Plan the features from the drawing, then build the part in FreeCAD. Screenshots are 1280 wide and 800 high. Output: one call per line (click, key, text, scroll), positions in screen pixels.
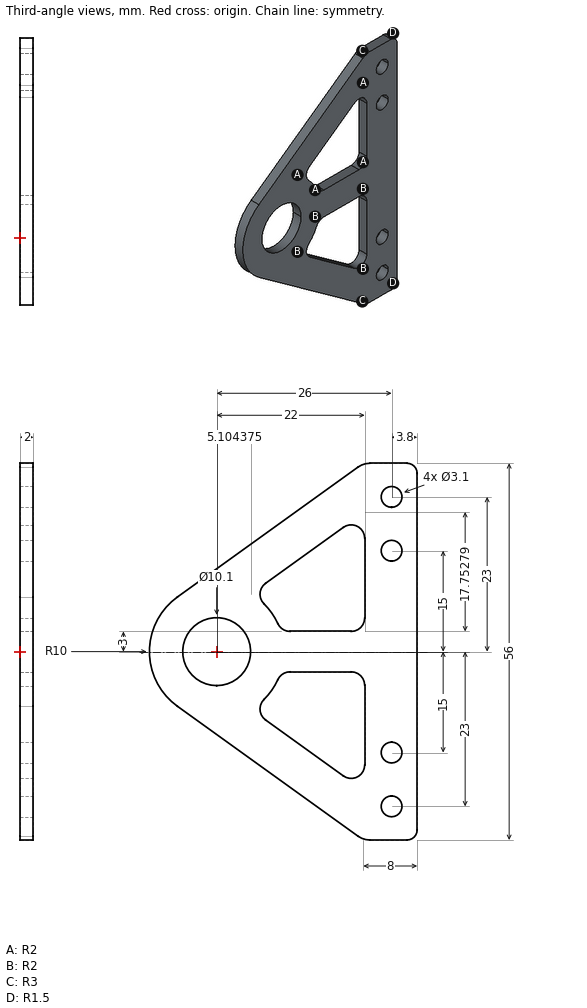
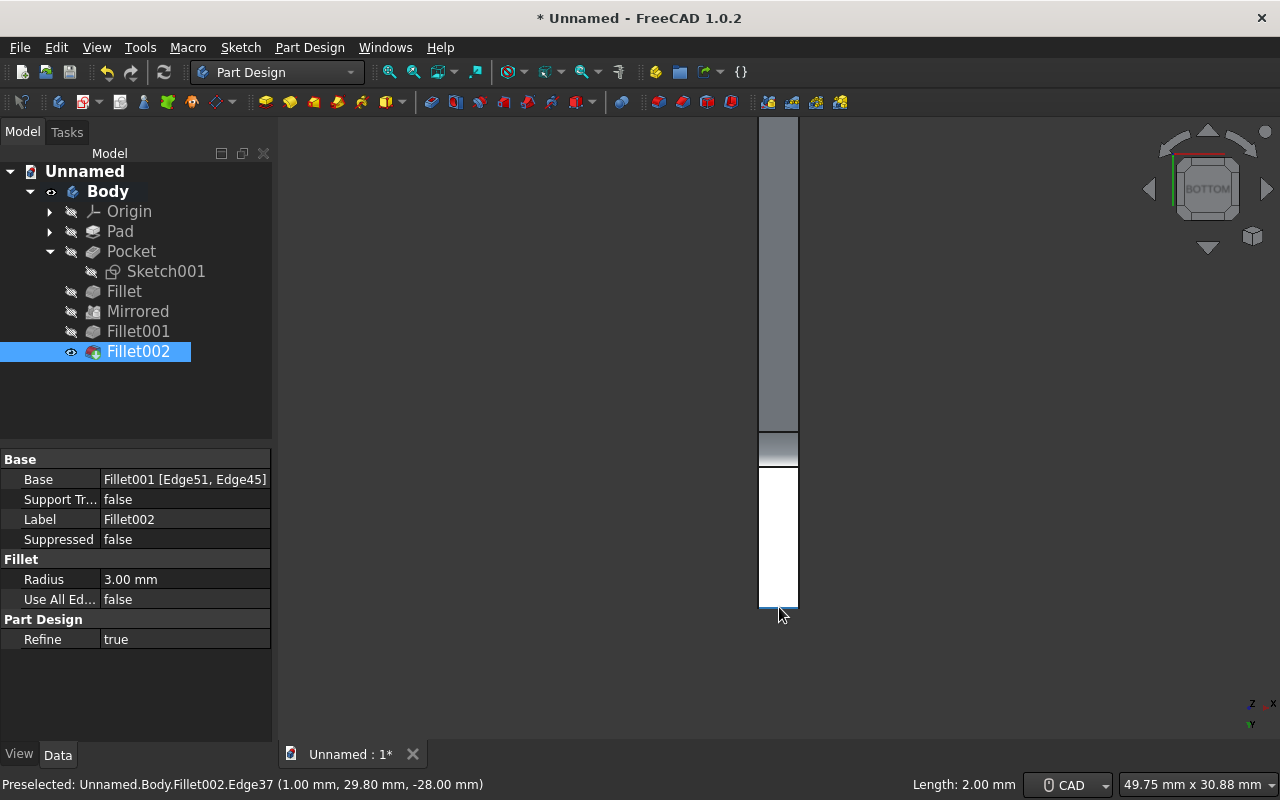
click(390, 72)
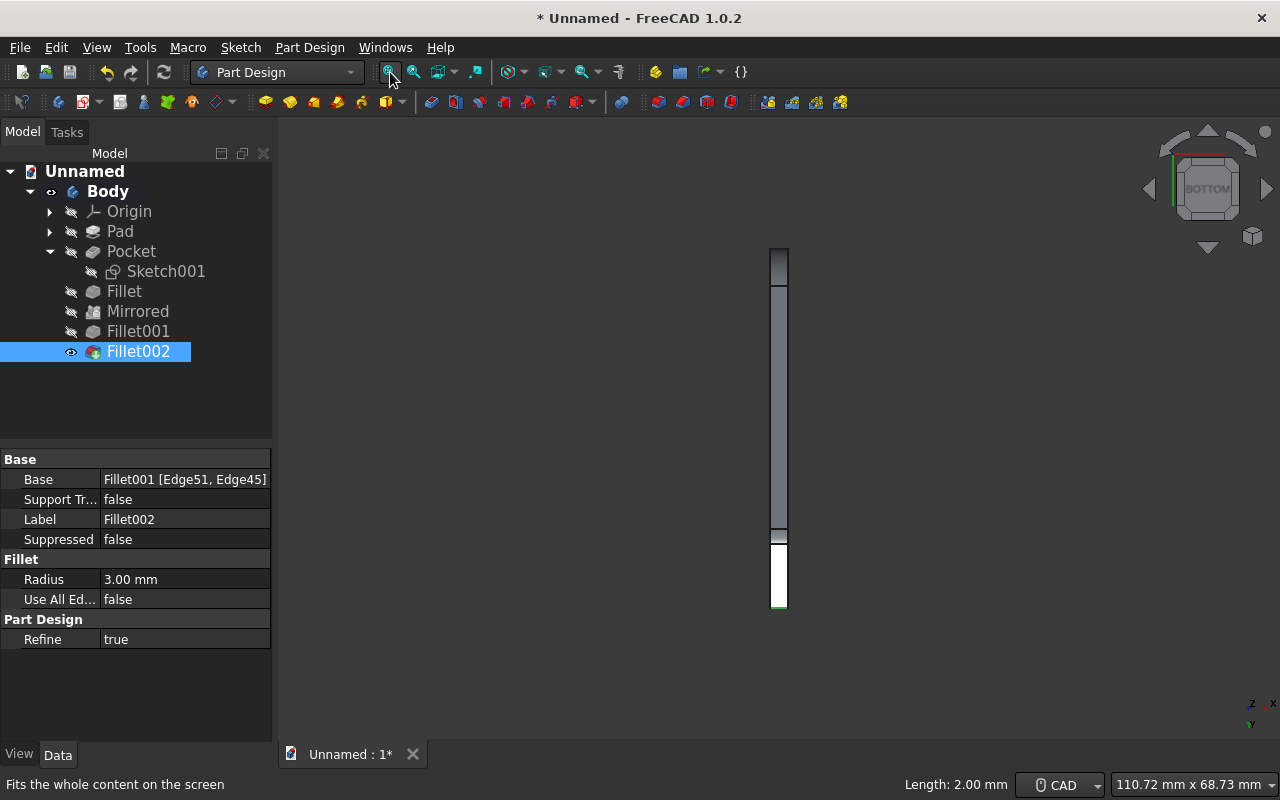
key(0)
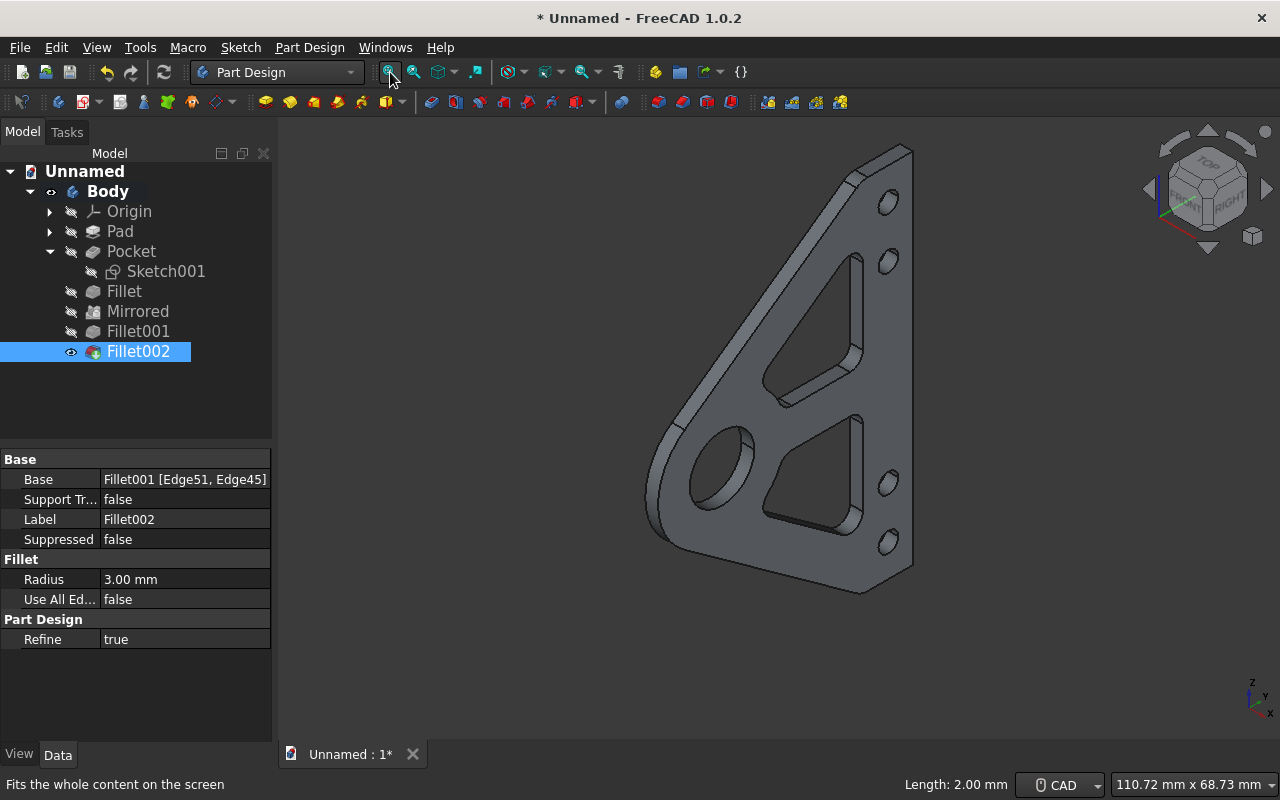
scroll(906, 147, up, 4)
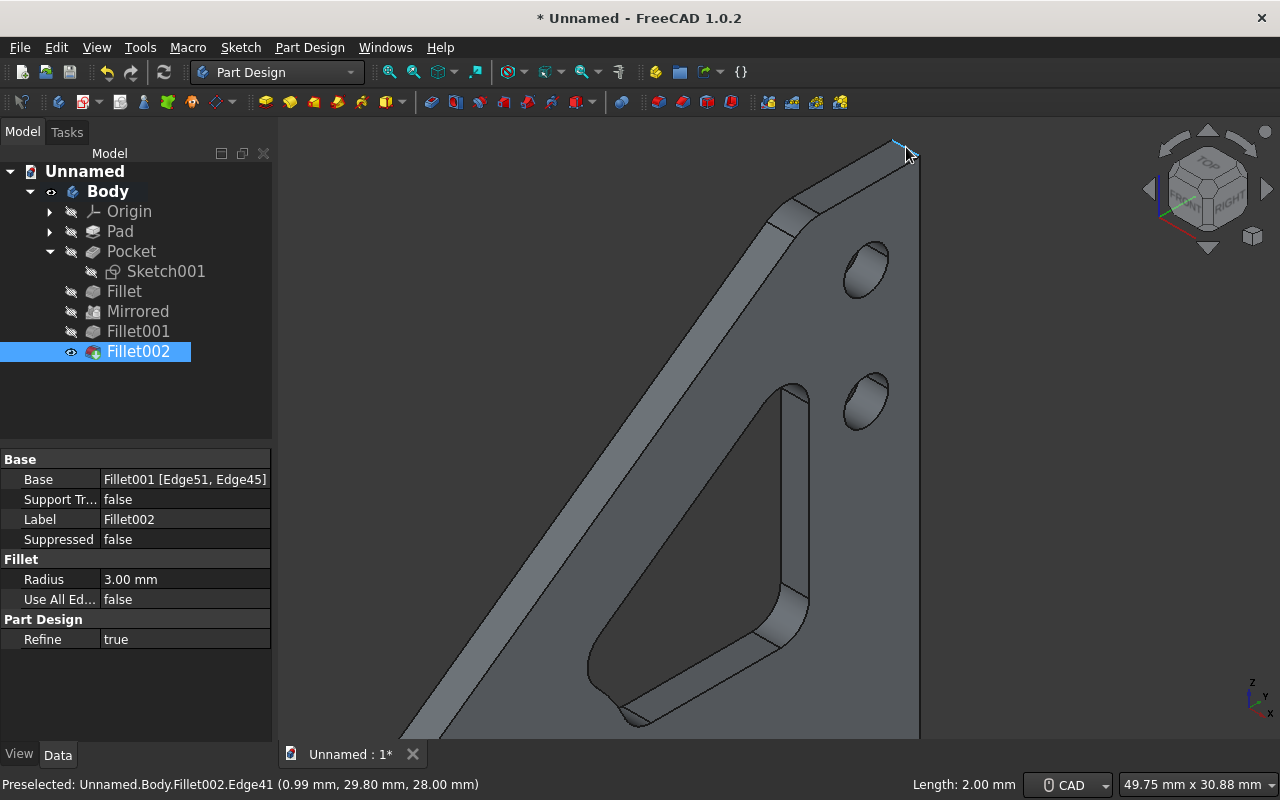
key(v)
key(f)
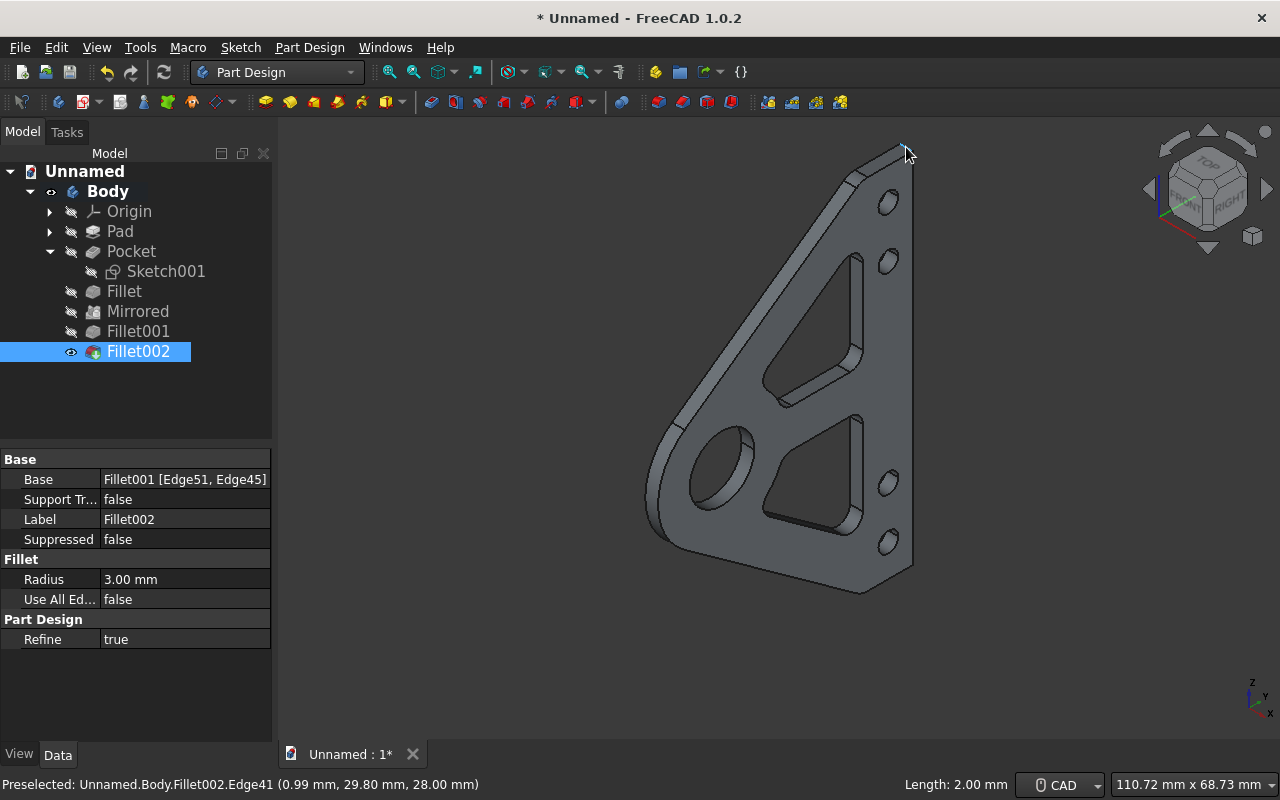
key(2)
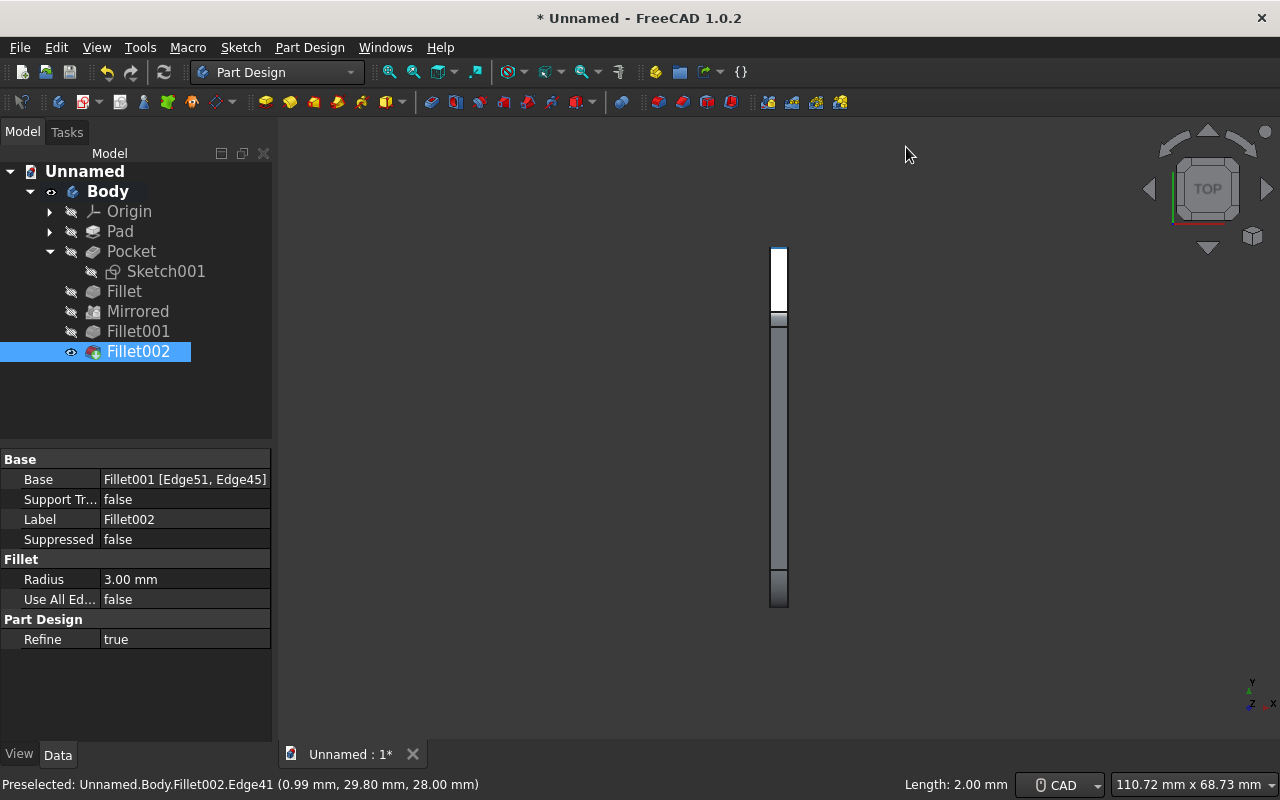
click(779, 247, ctrl)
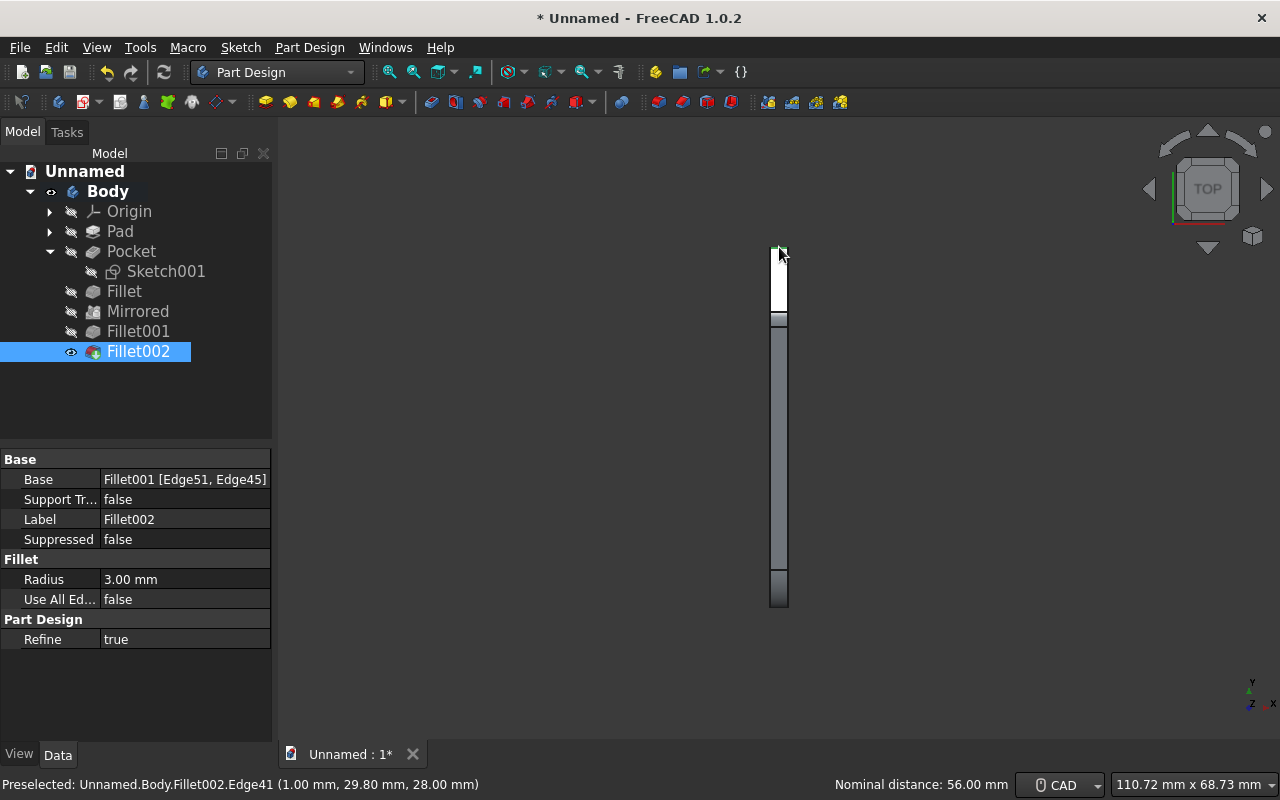
click(660, 102)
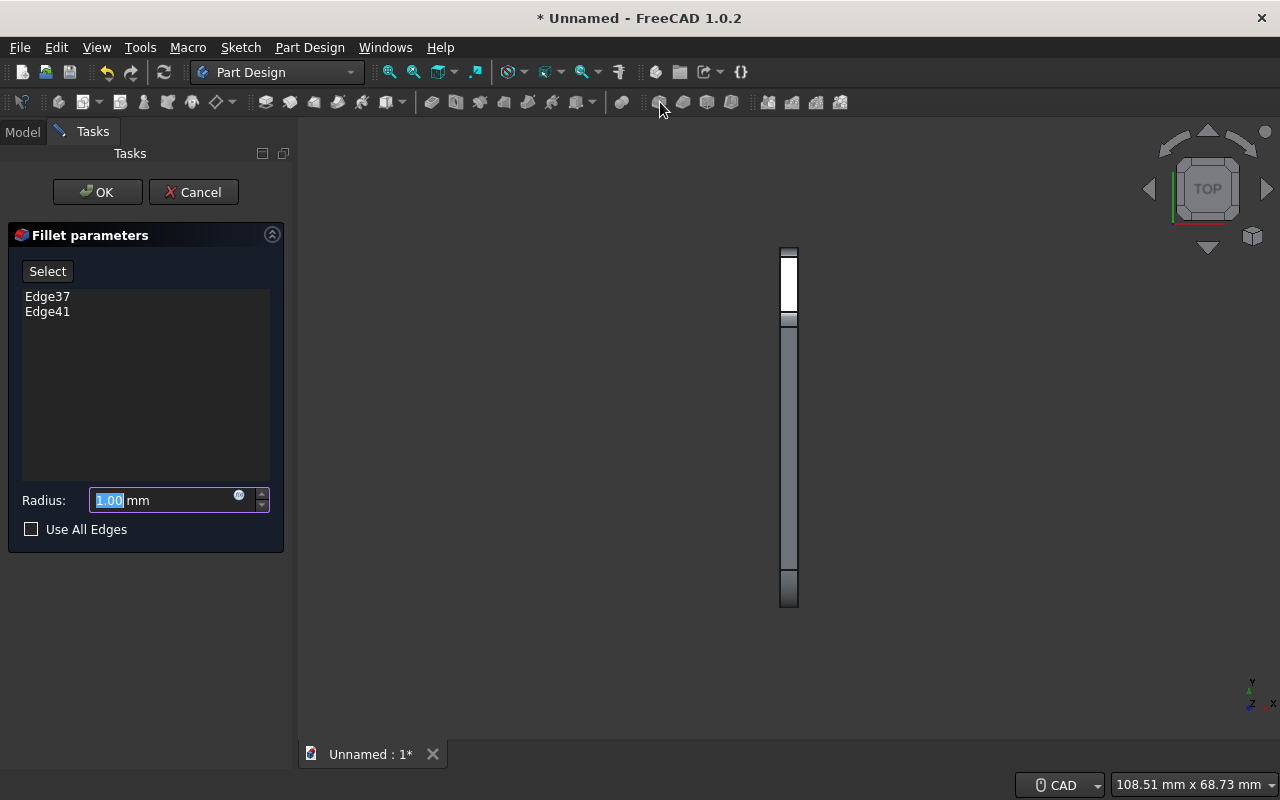
text(1.5)
key(Tab)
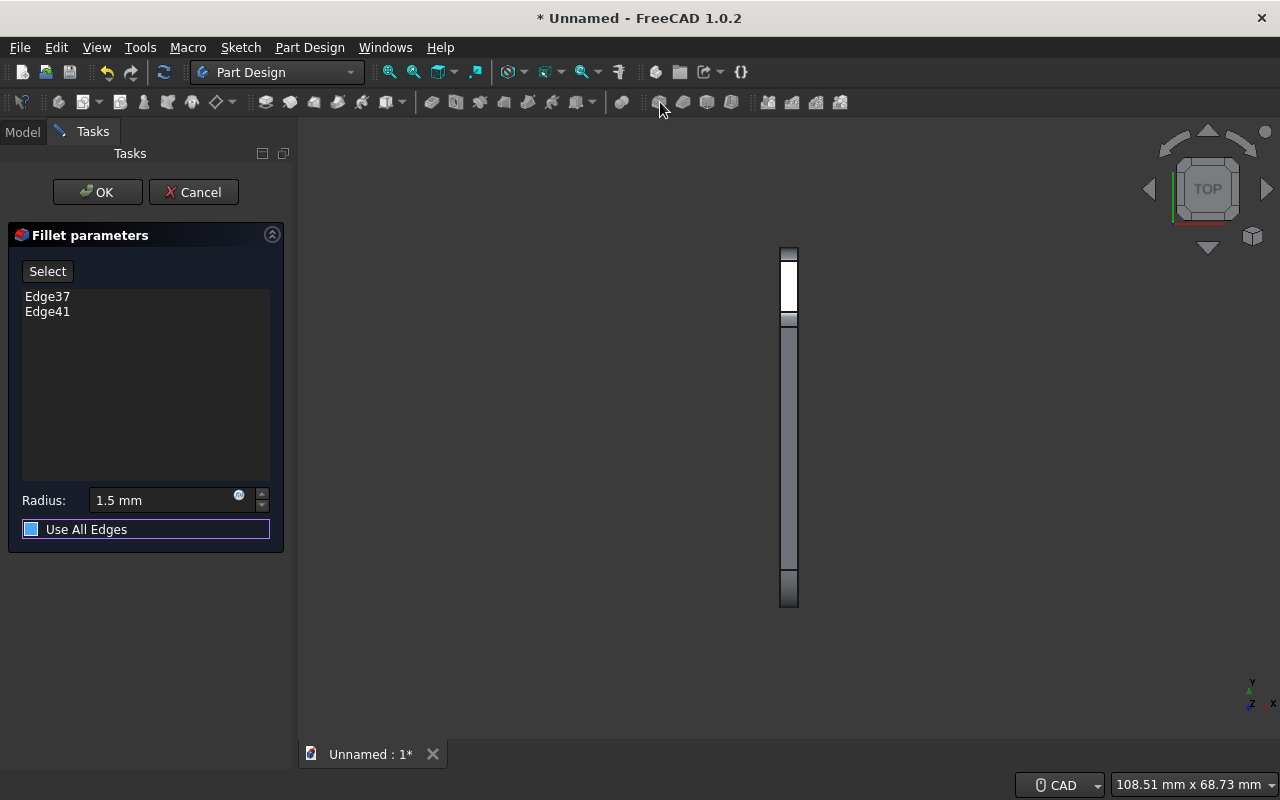
click(98, 192)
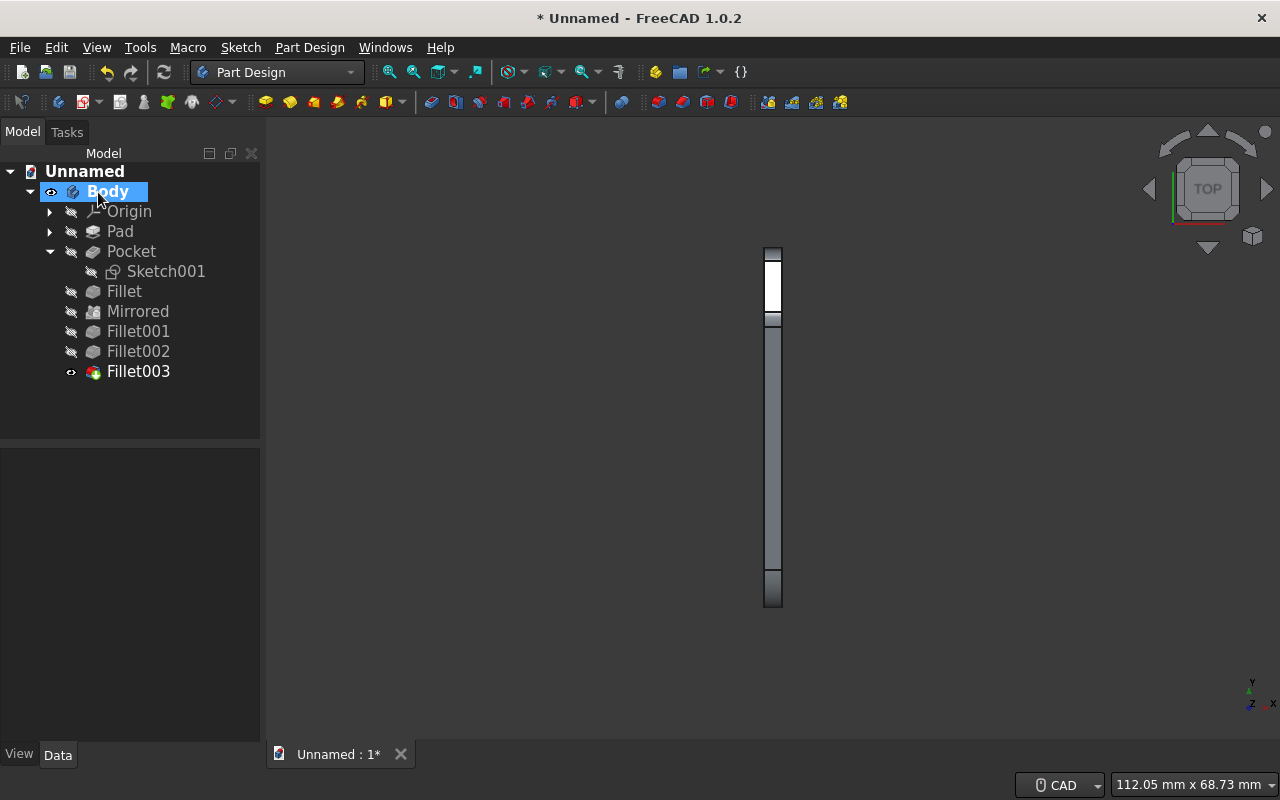
key(0)